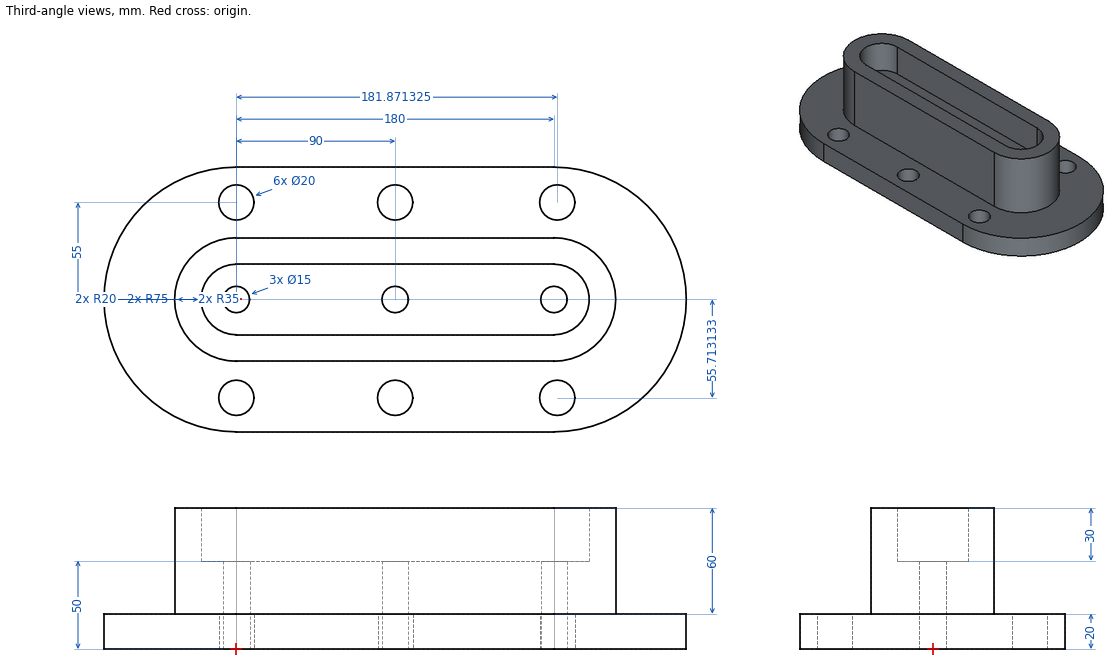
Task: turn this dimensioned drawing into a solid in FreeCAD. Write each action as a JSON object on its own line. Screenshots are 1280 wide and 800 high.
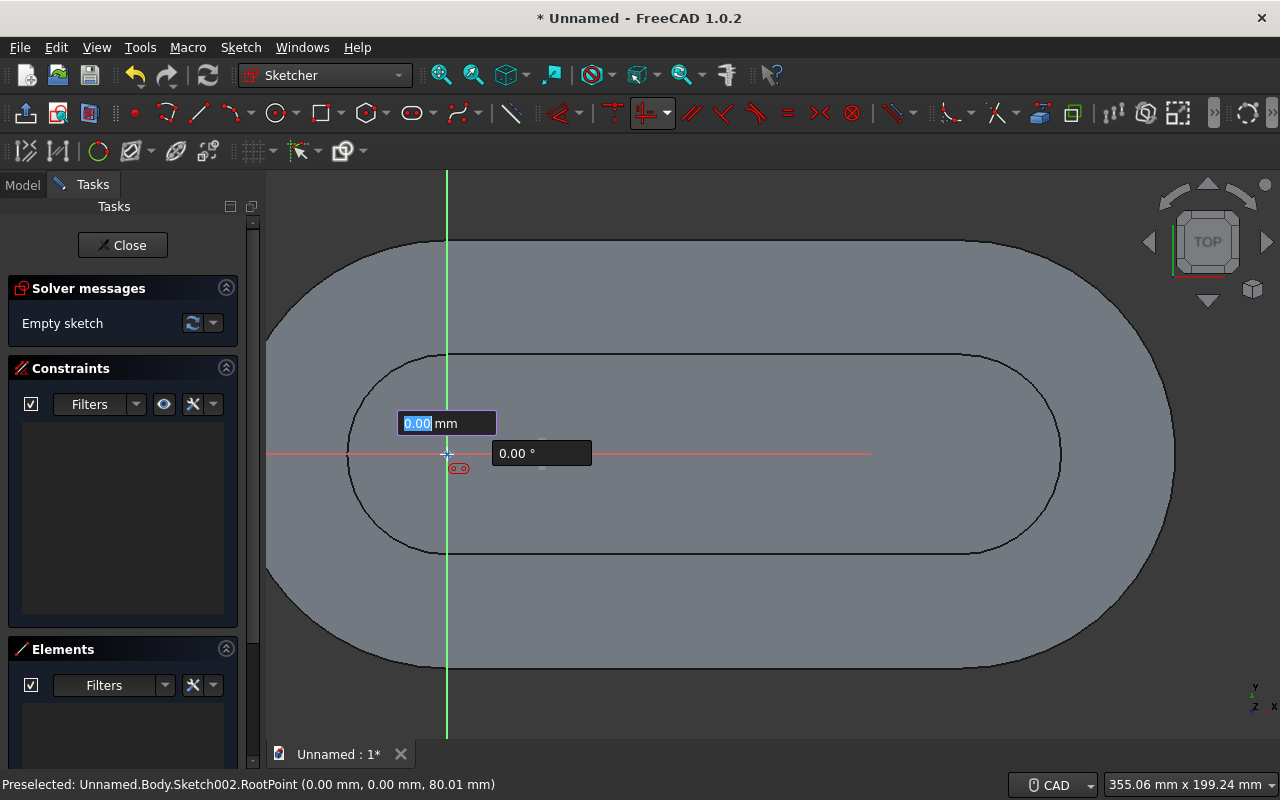
{"action": "left_click", "coordinate": [961, 445]}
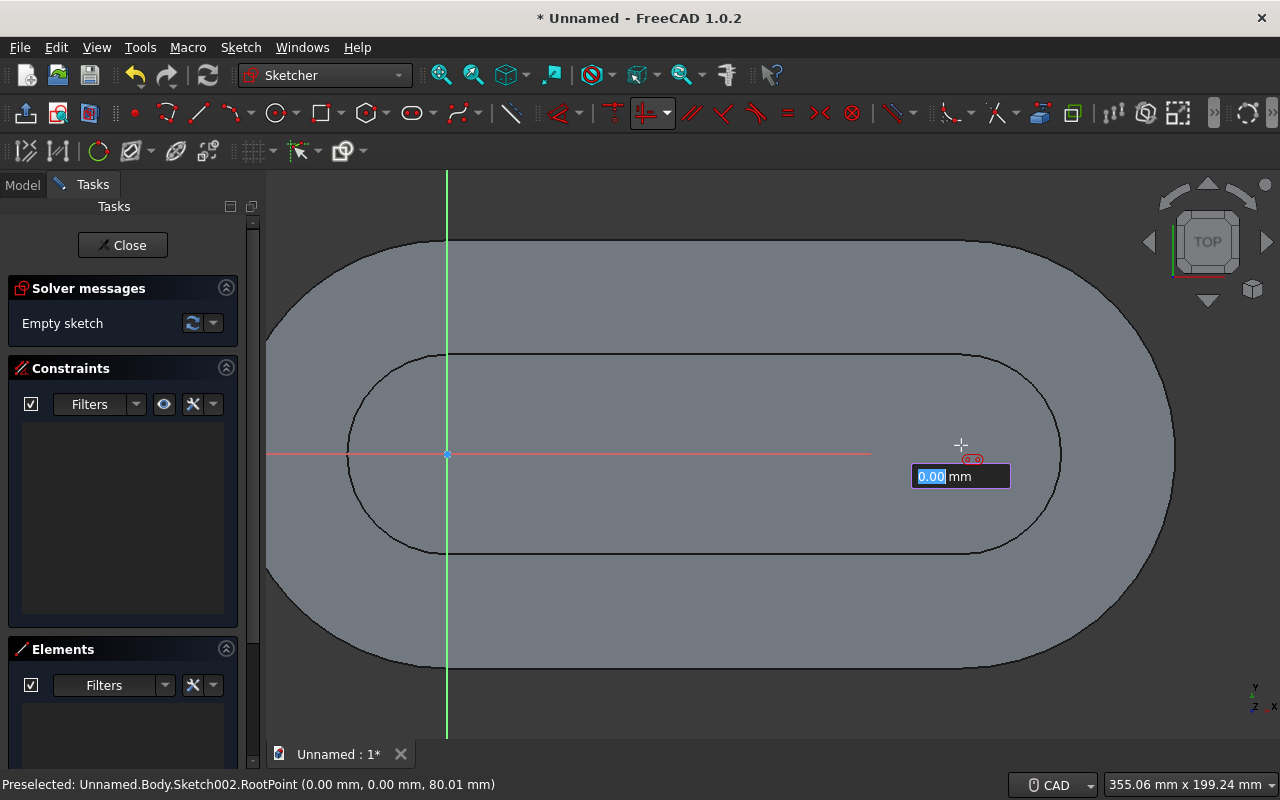
{"action": "left_click", "coordinate": [704, 397]}
{"action": "key", "text": "Escape"}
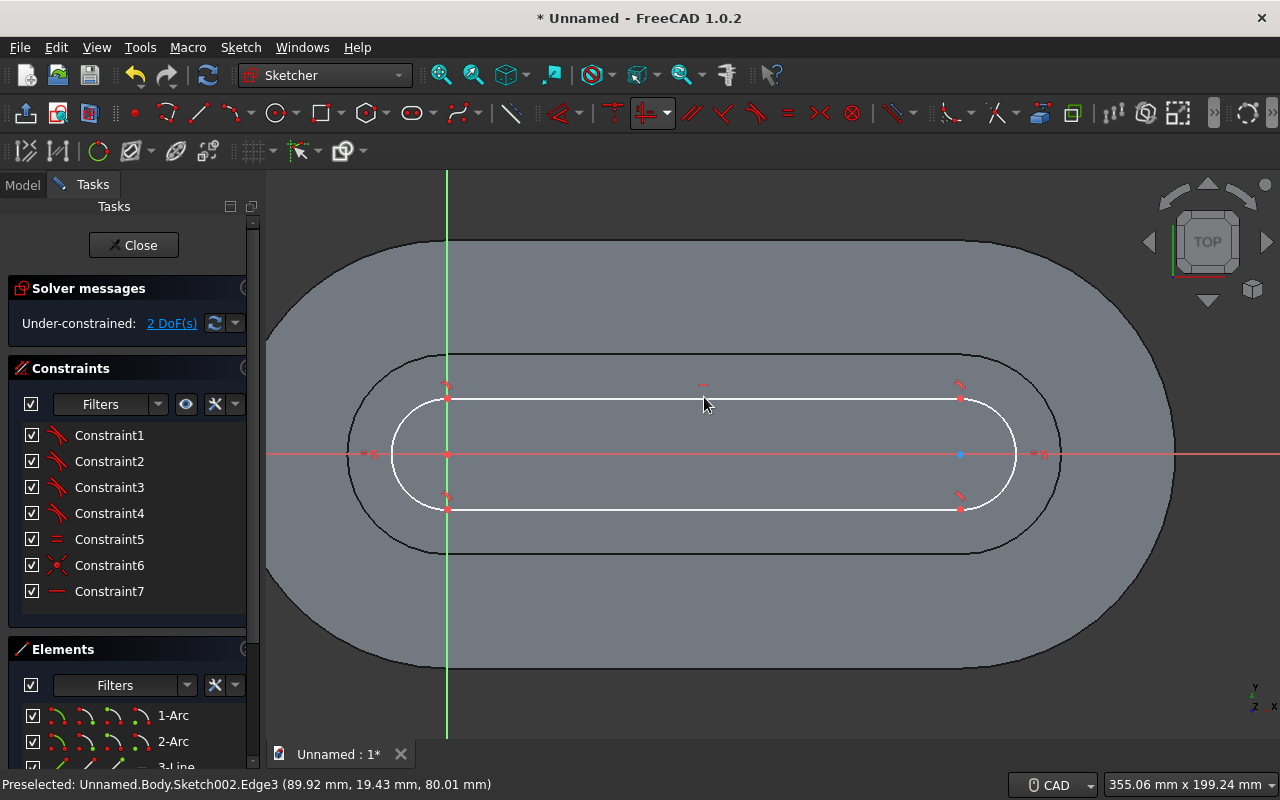
{"action": "left_click", "coordinate": [558, 114]}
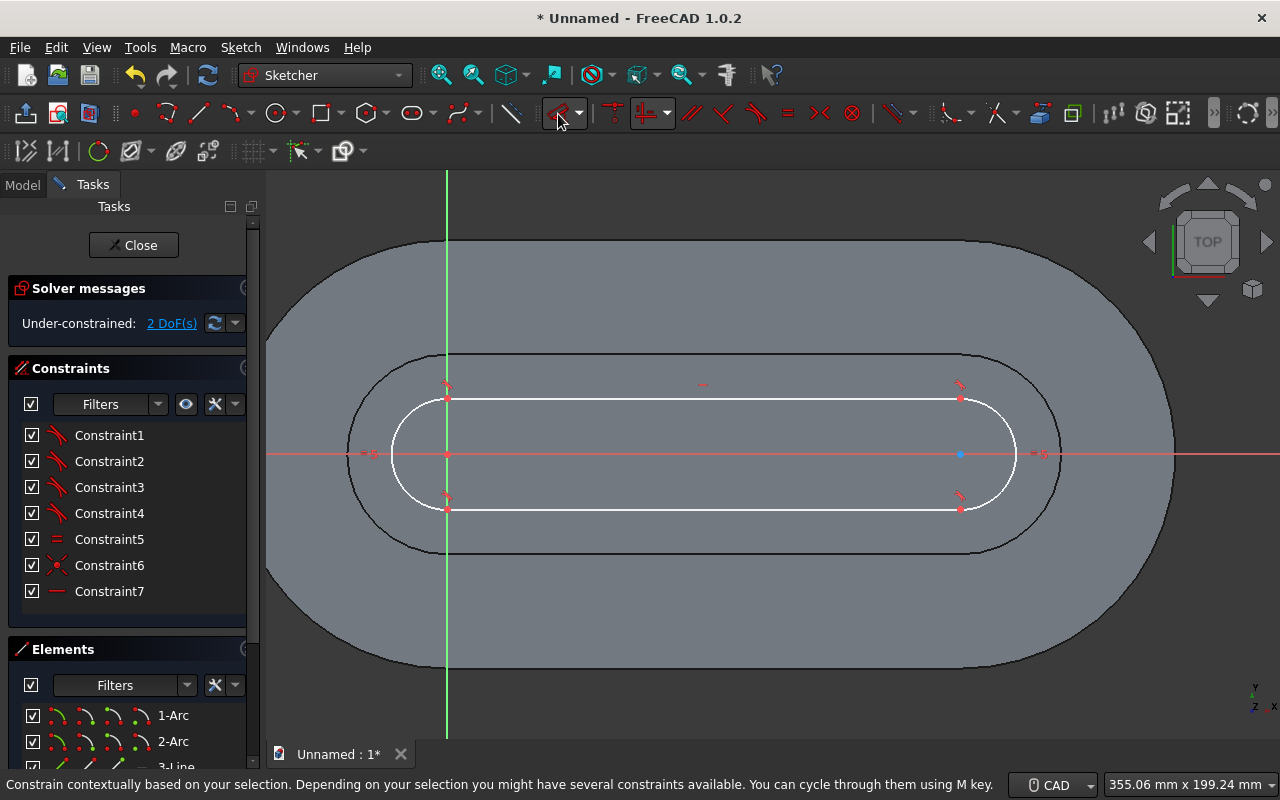
{"action": "left_click", "coordinate": [402, 422]}
{"action": "left_click", "coordinate": [376, 403]}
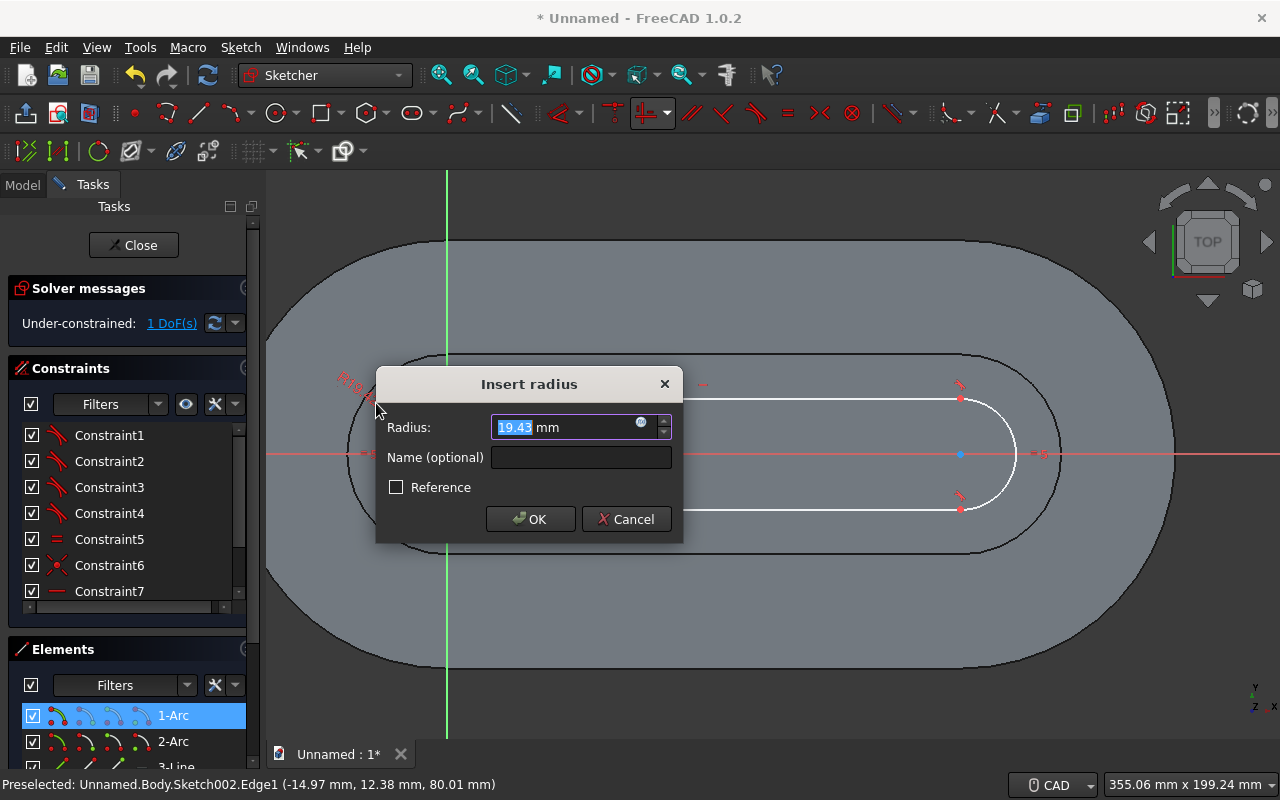
{"action": "type", "text": "20"}
{"action": "key", "text": "Return"}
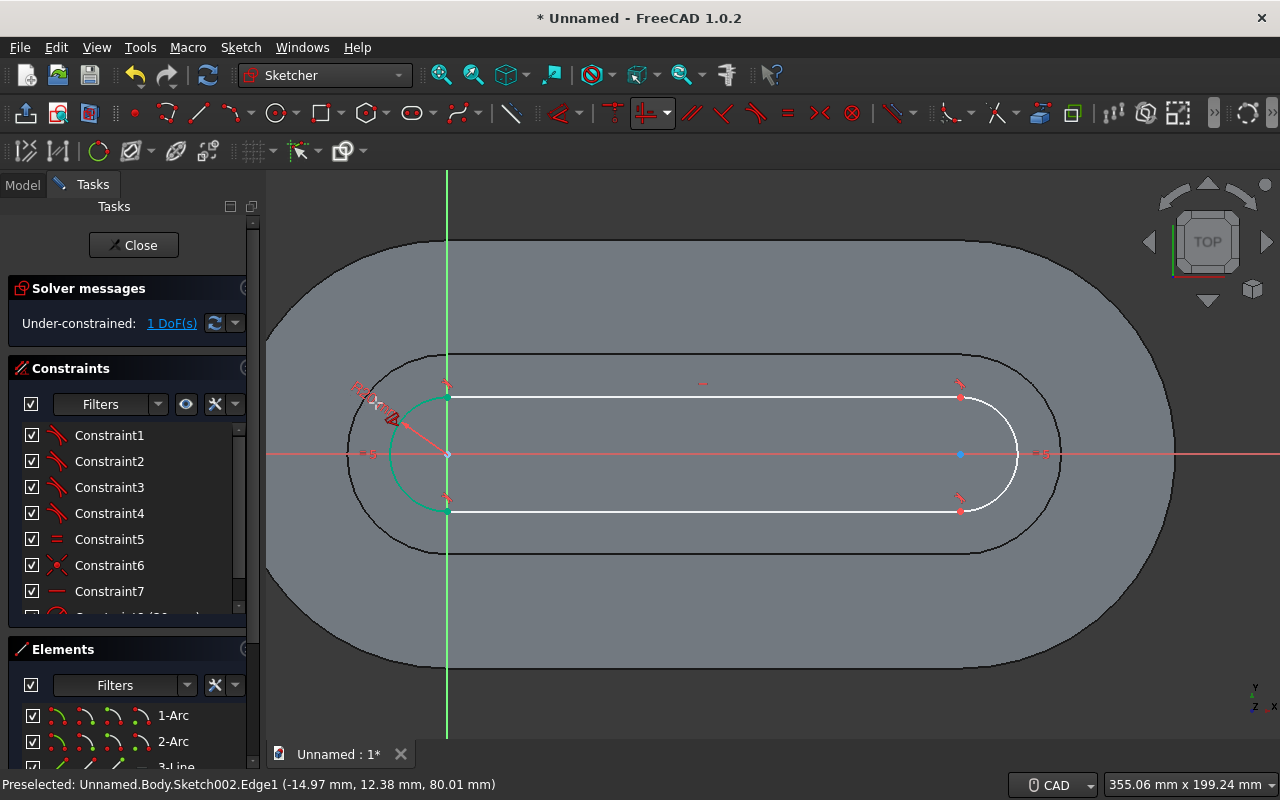
{"action": "left_click", "coordinate": [601, 397]}
{"action": "left_click", "coordinate": [704, 363]}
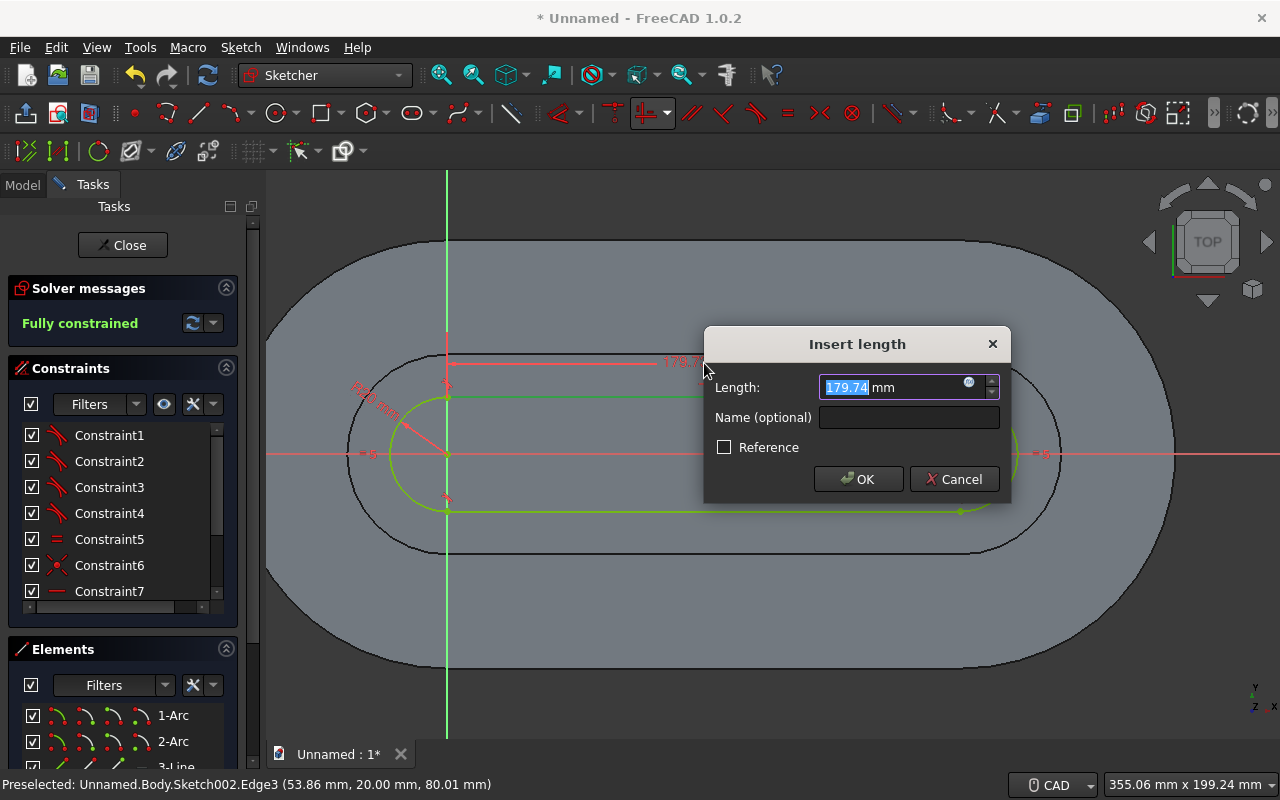
{"action": "type", "text": "180"}
{"action": "key", "text": "Return"}
{"action": "key", "text": "Escape"}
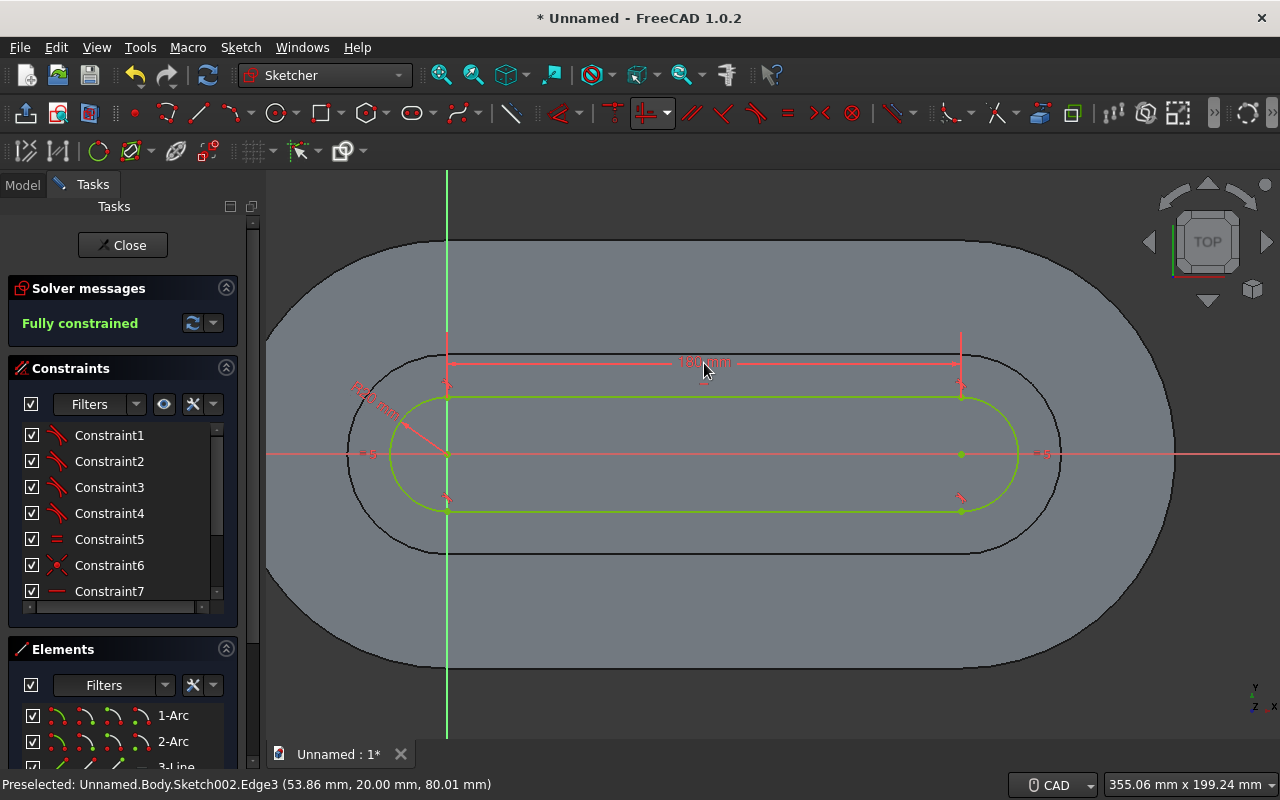
{"action": "left_click", "coordinate": [123, 245]}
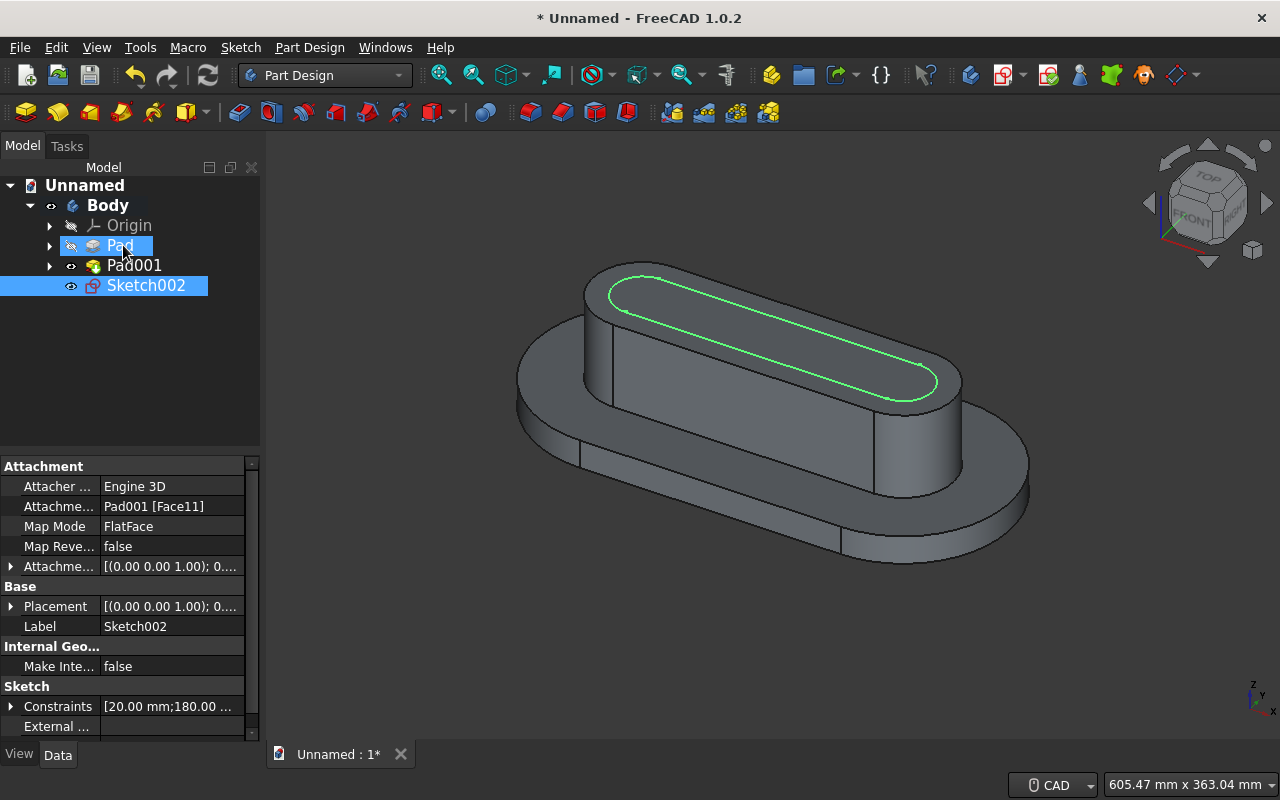
{"action": "left_click", "coordinate": [240, 112]}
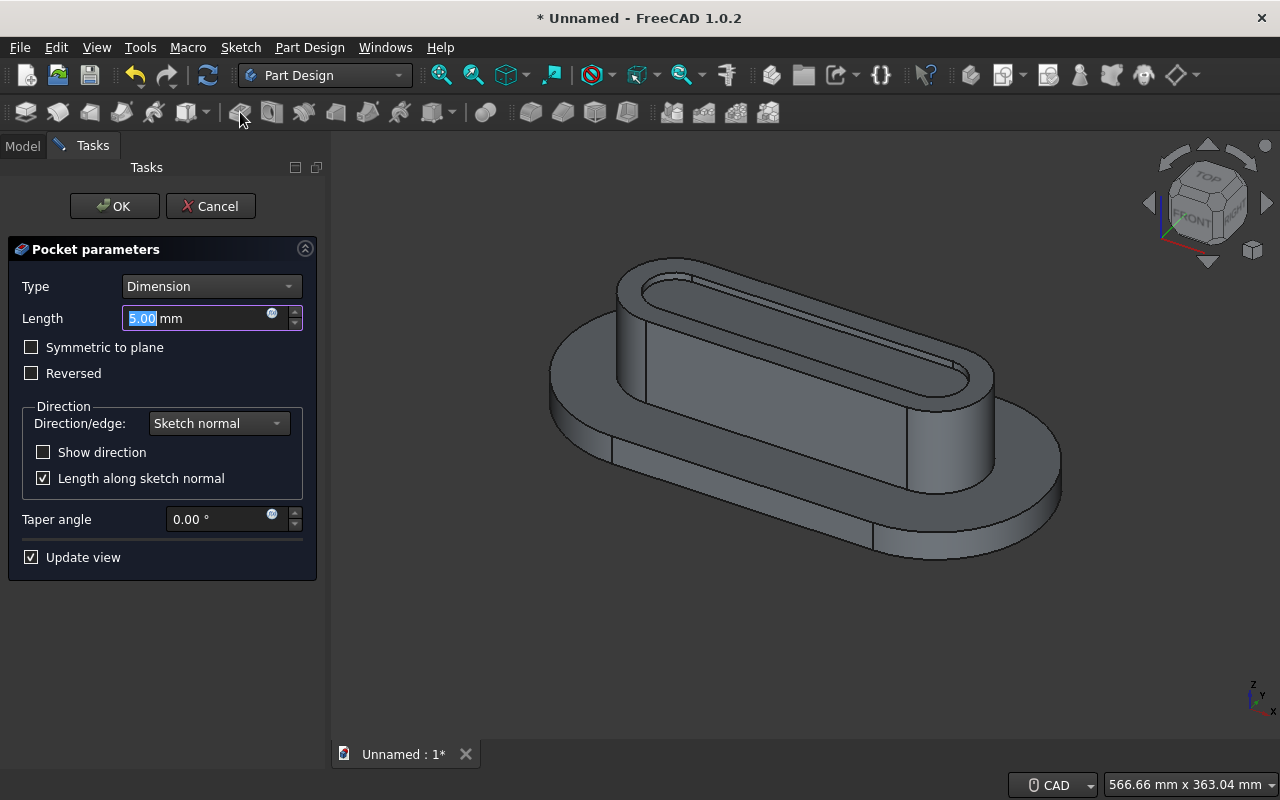
{"action": "type", "text": "30"}
{"action": "key", "text": "Tab"}